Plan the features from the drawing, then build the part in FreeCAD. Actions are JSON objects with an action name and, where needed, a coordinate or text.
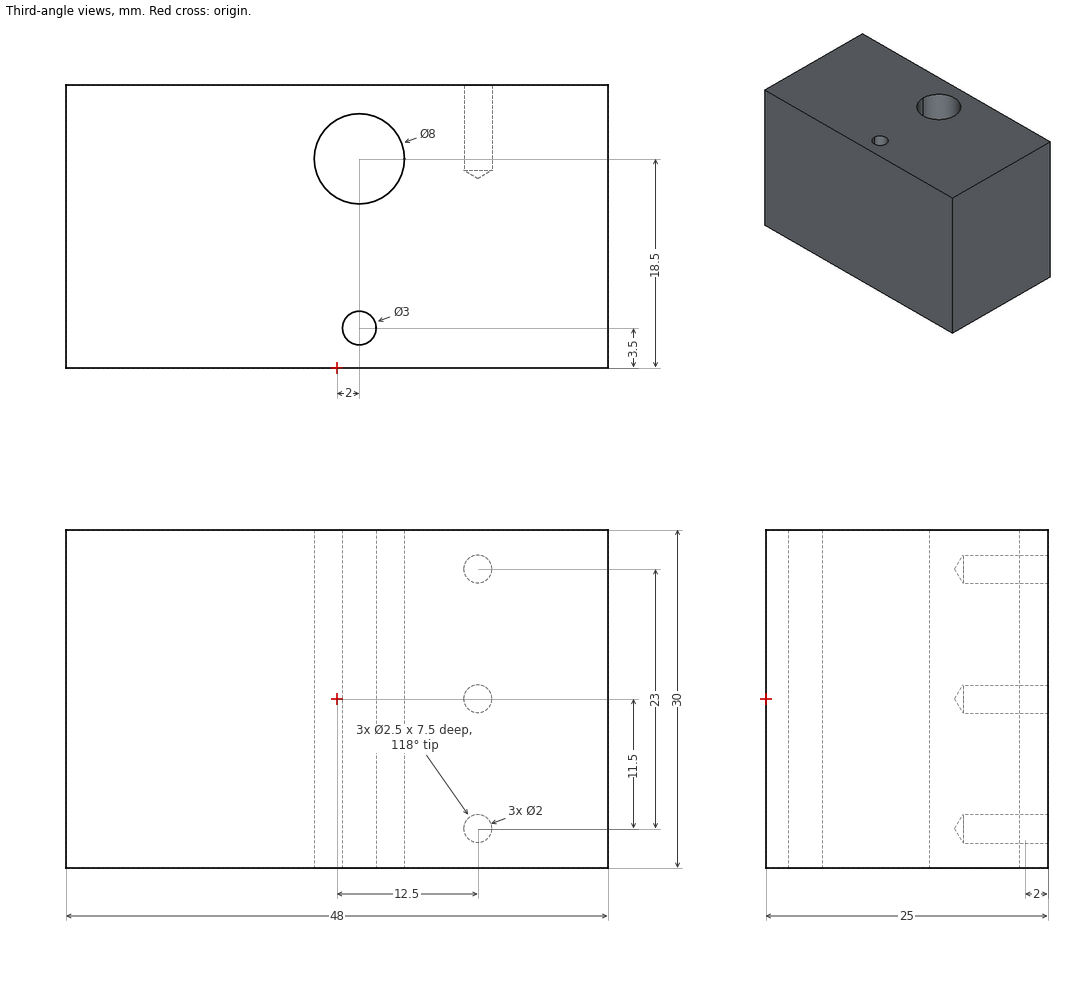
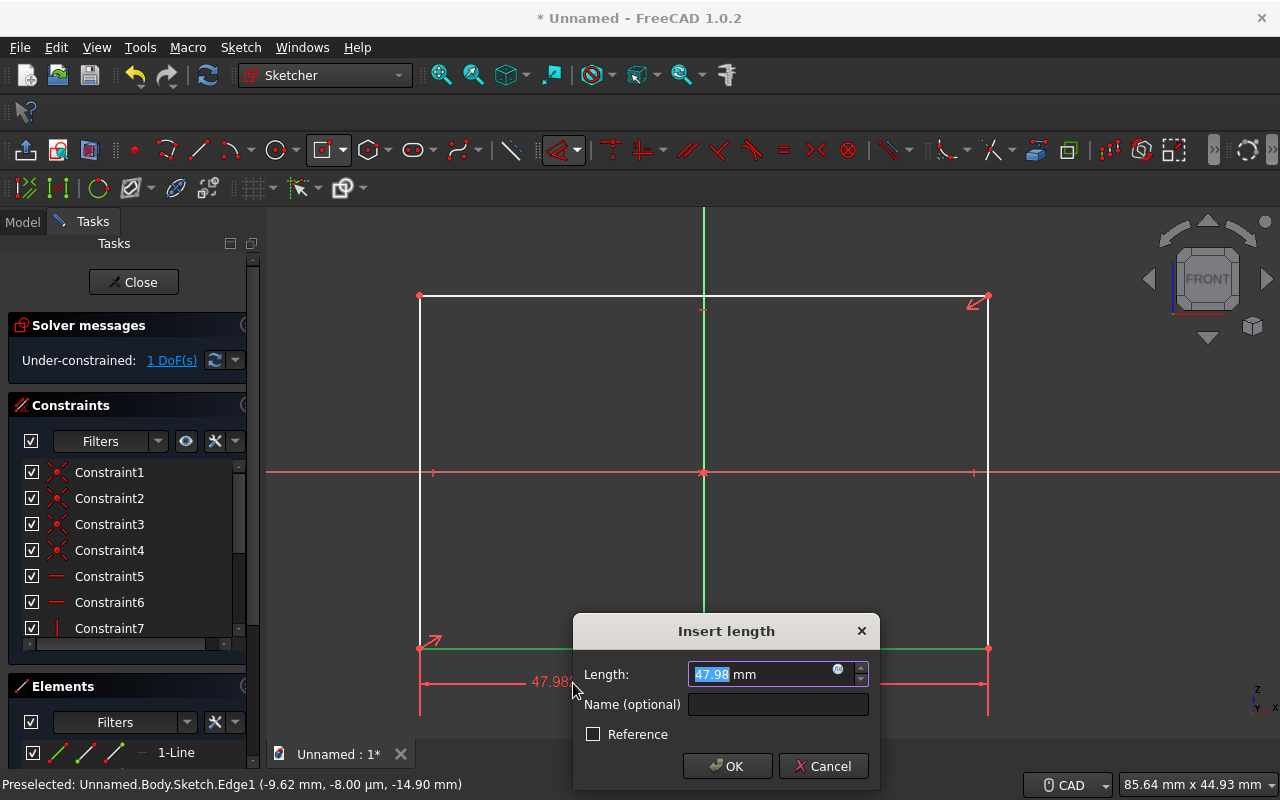
{"action": "type", "text": "48"}
{"action": "key", "text": "Return"}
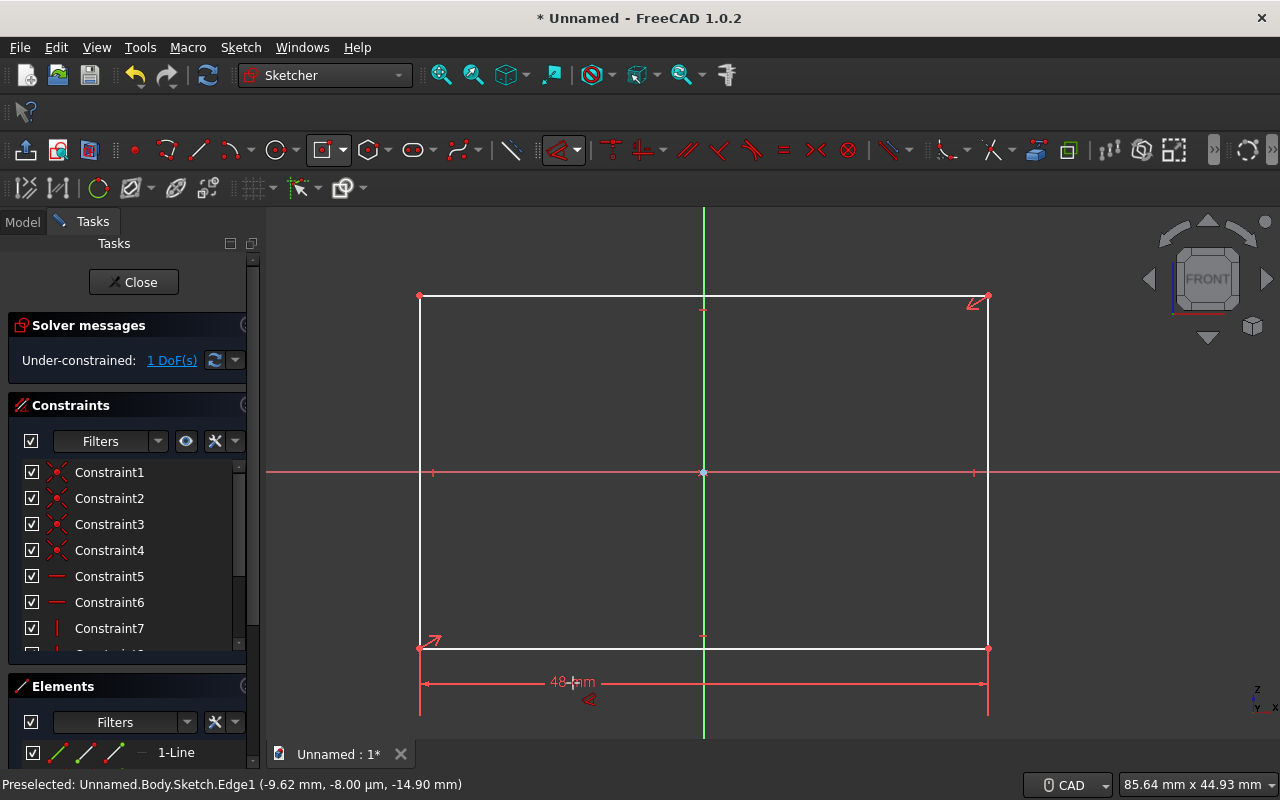
{"action": "left_click", "coordinate": [988, 543]}
{"action": "left_click", "coordinate": [1022, 391]}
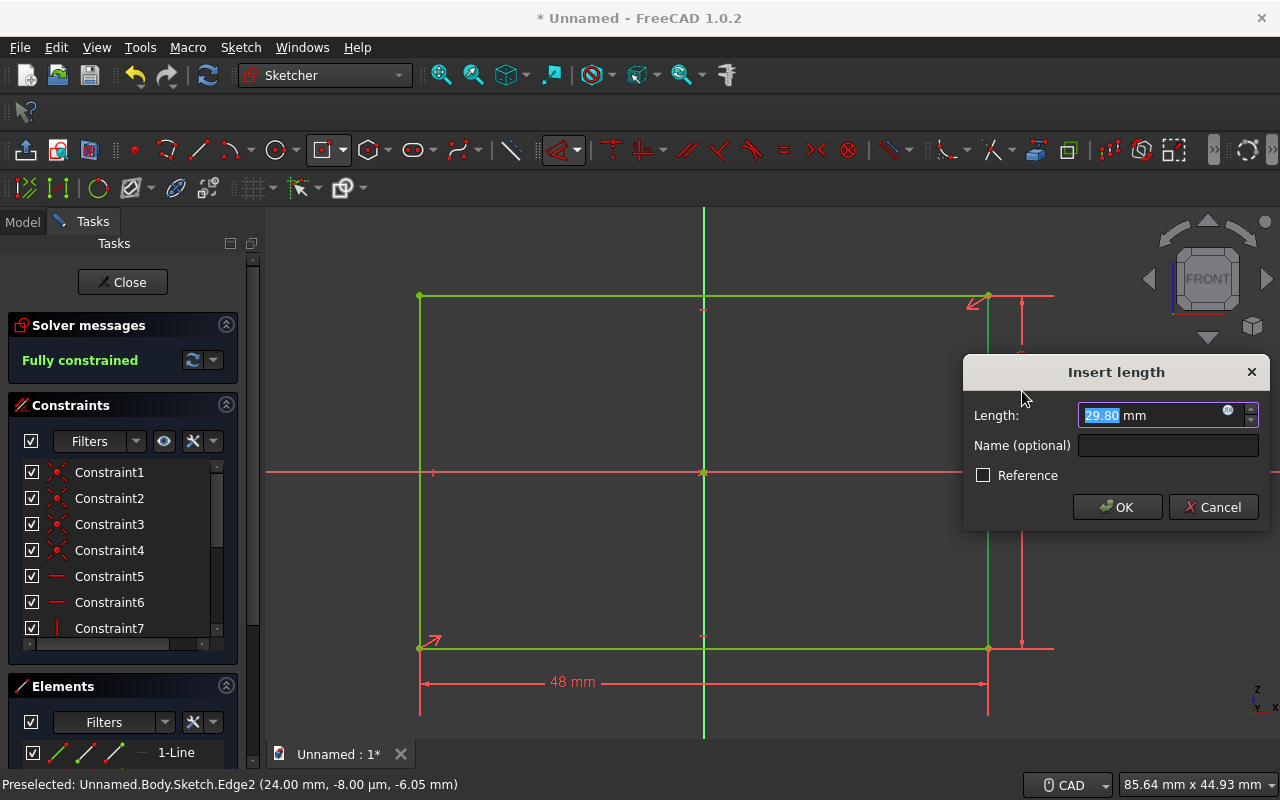
{"action": "type", "text": "30"}
{"action": "key", "text": "Return"}
{"action": "key", "text": "Escape"}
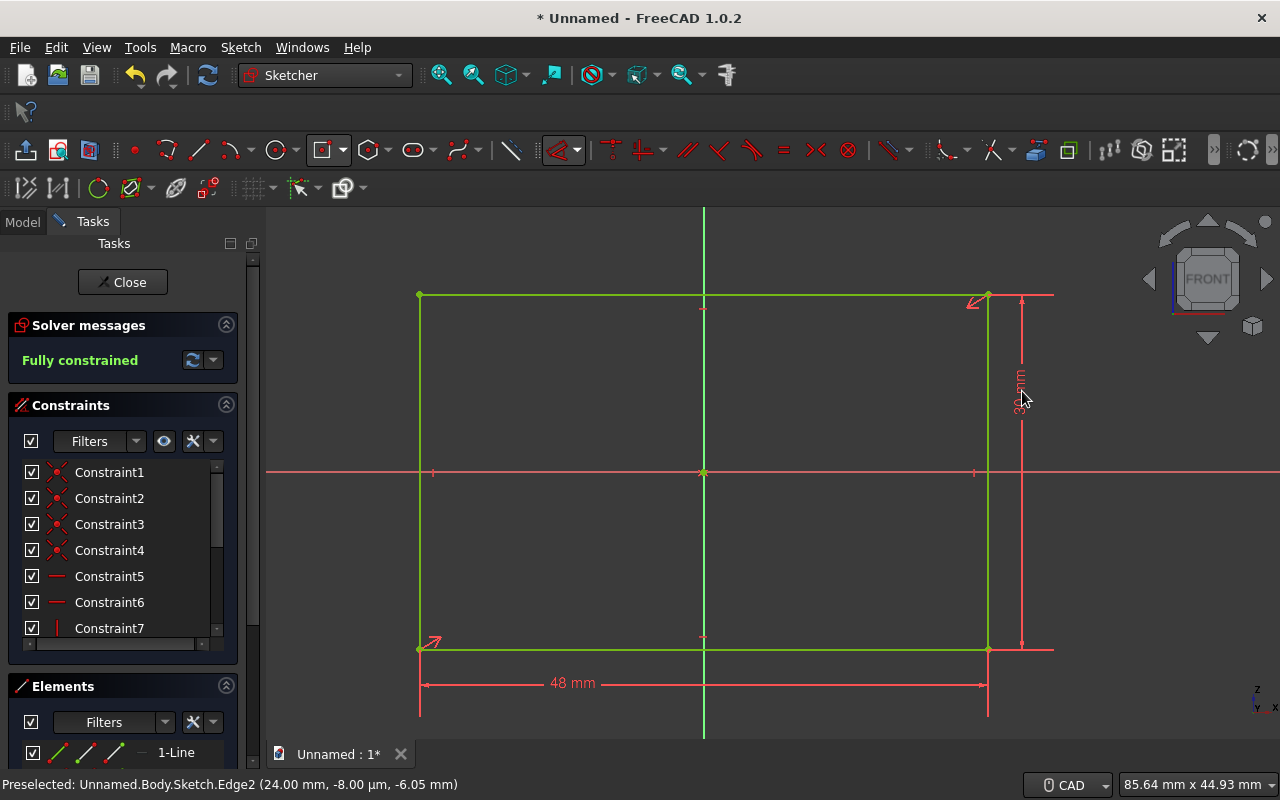
{"action": "left_click", "coordinate": [123, 282]}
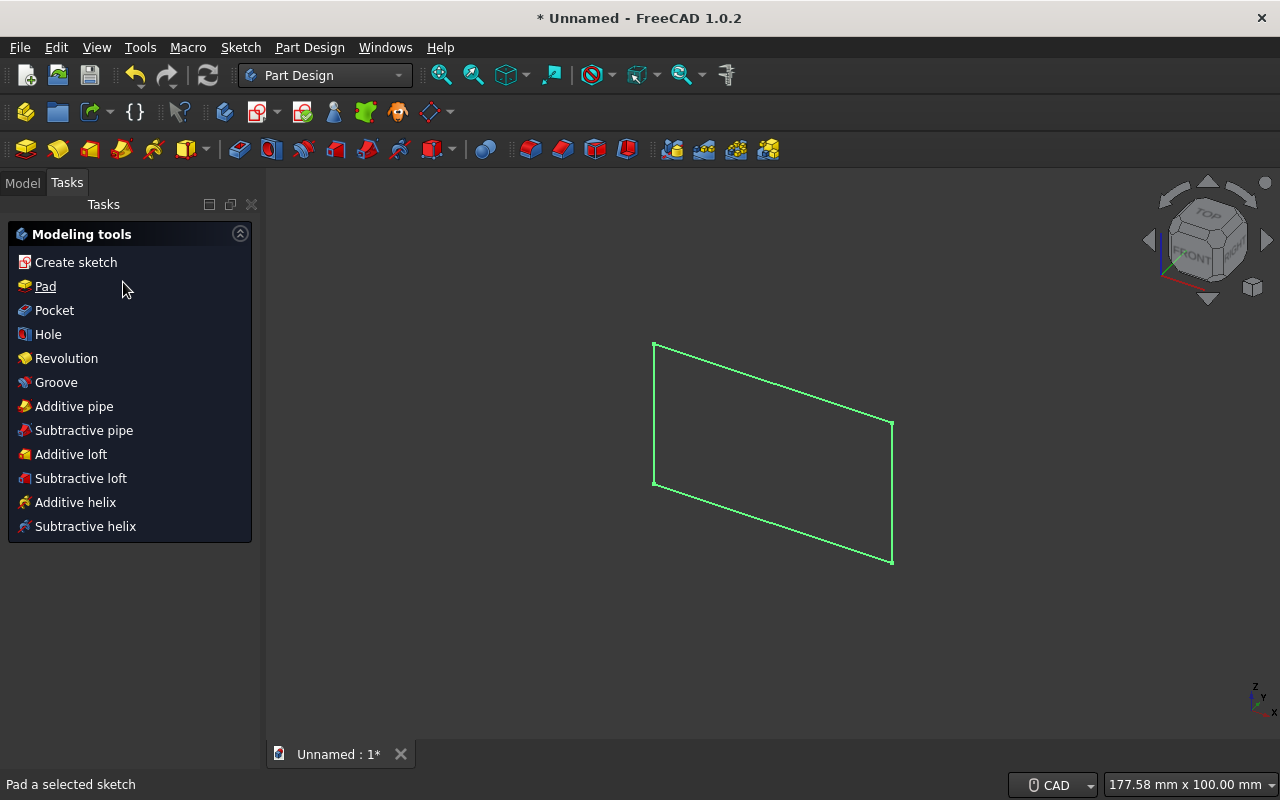
{"action": "left_click", "coordinate": [26, 150]}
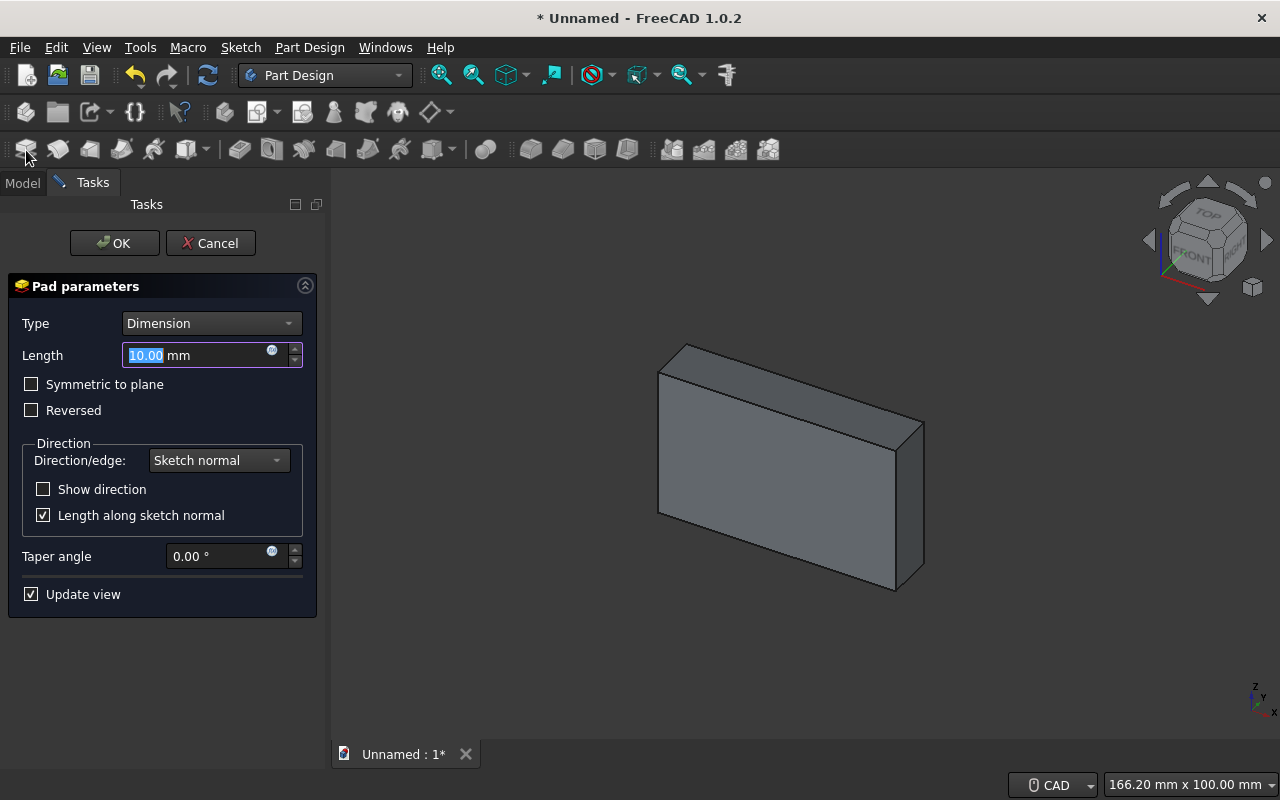
{"action": "type", "text": "25"}
{"action": "key", "text": "Tab"}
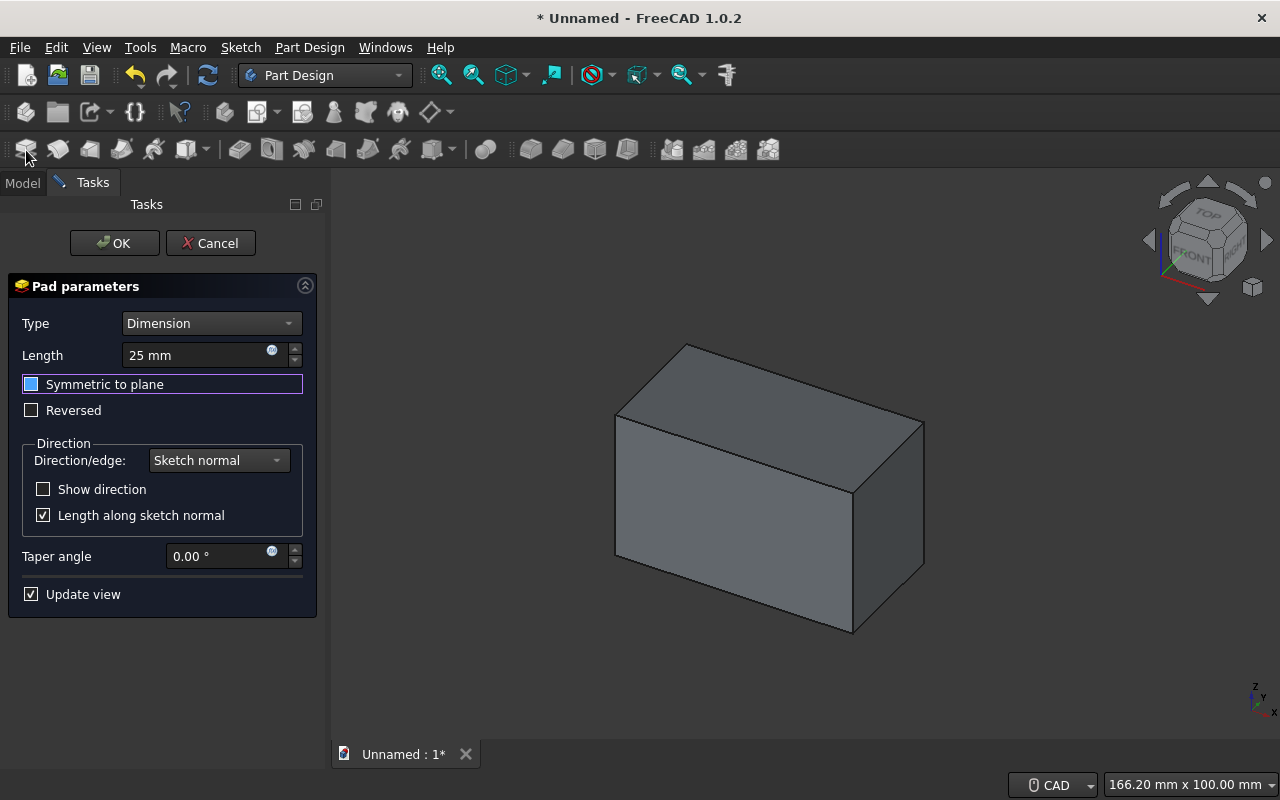
{"action": "left_click", "coordinate": [30, 410]}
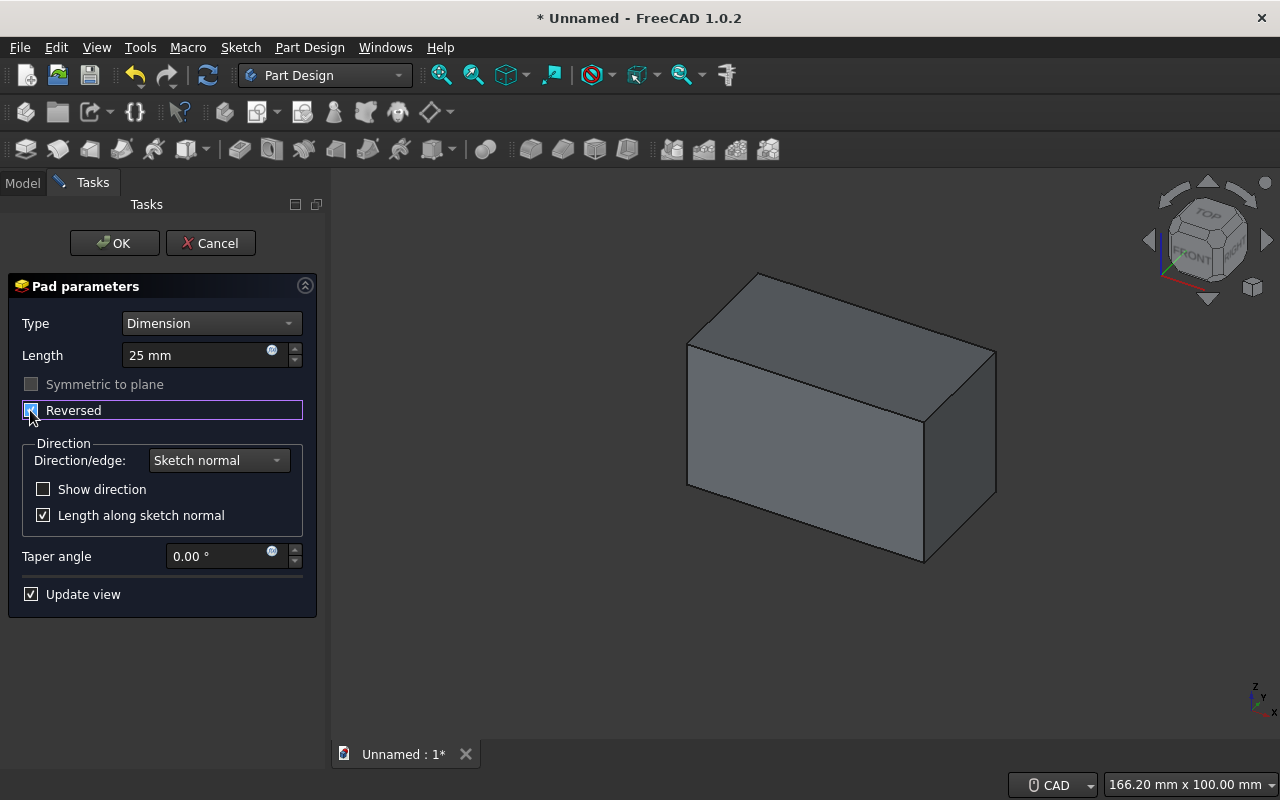
{"action": "left_click", "coordinate": [115, 243]}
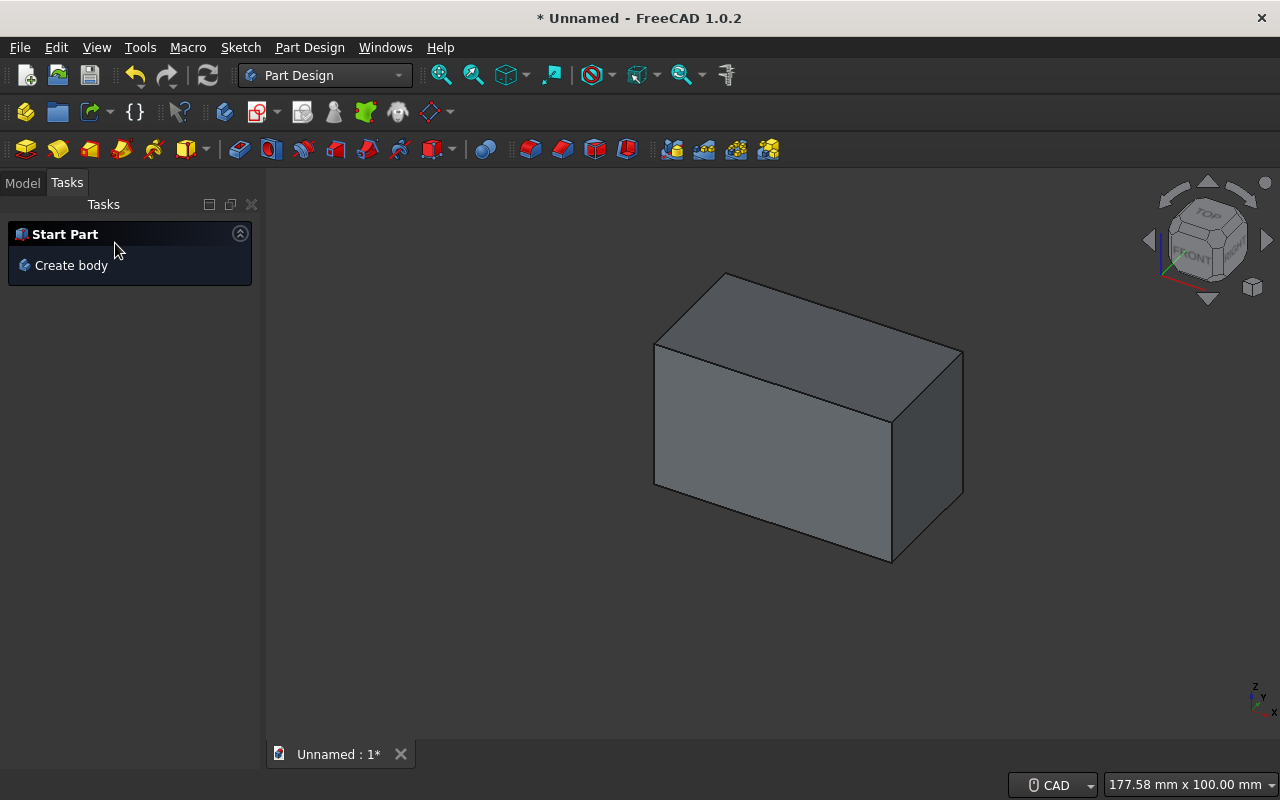
{"action": "left_click", "coordinate": [843, 358]}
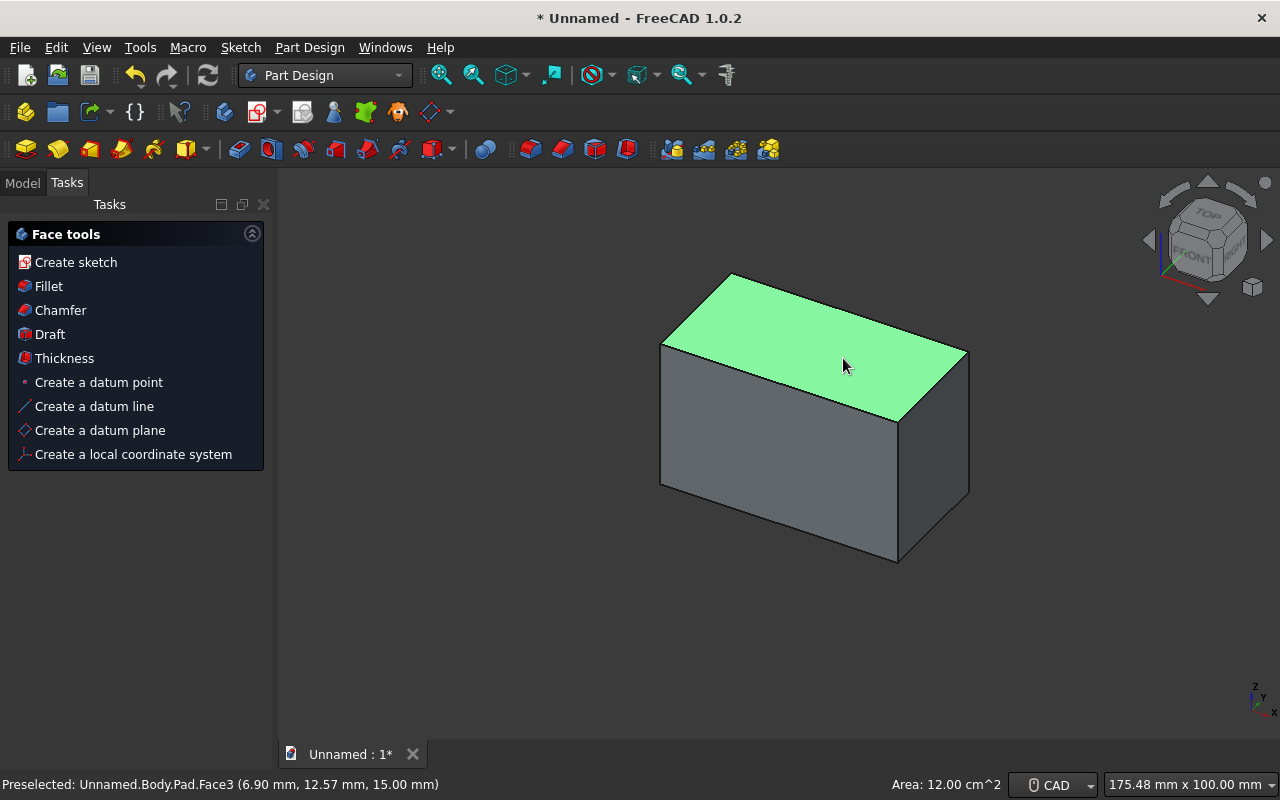
{"action": "left_click", "coordinate": [258, 112]}